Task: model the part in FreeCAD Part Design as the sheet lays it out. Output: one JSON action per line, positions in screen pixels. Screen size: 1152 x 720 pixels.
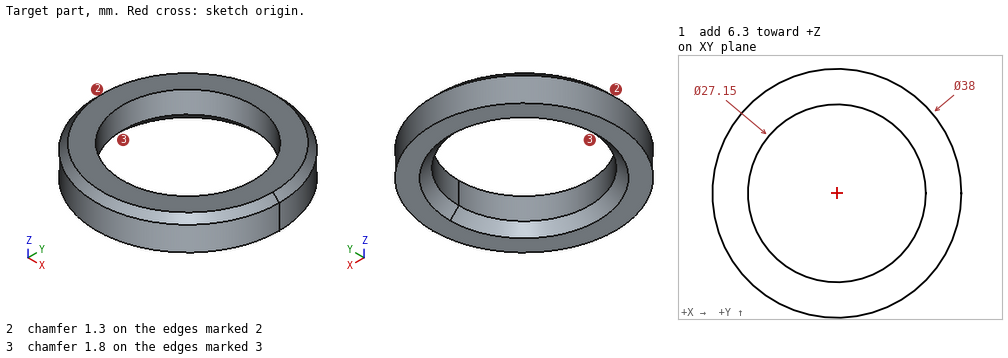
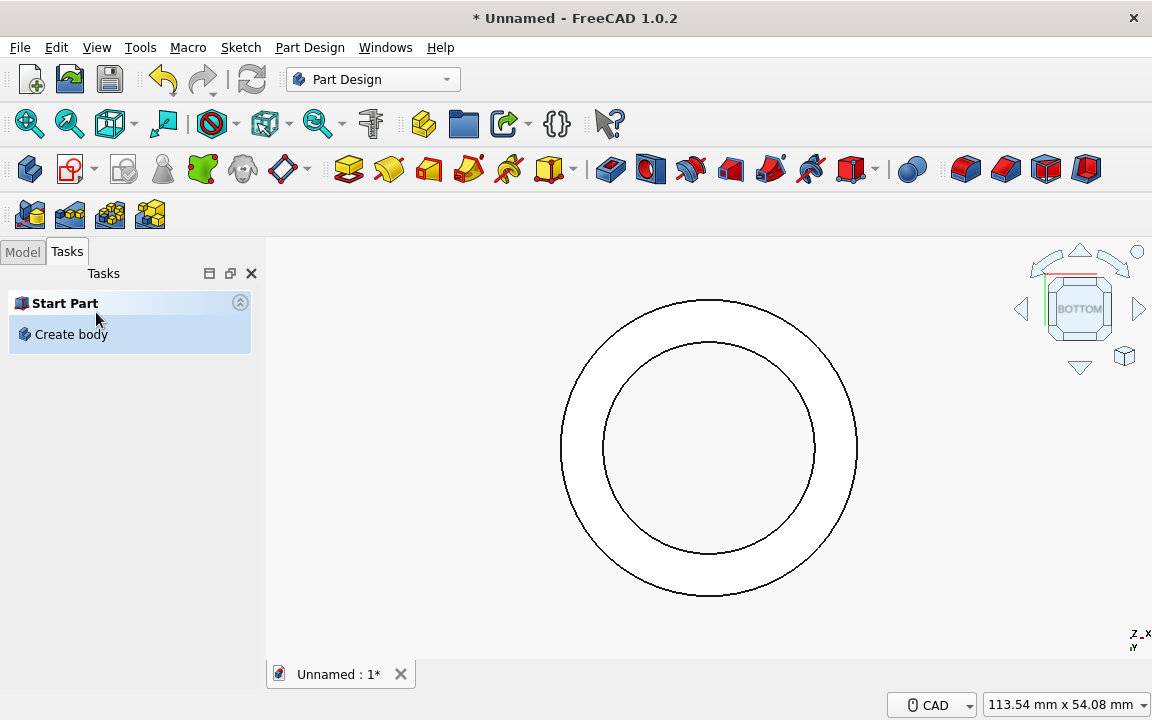
{"action": "left_click", "coordinate": [676, 548]}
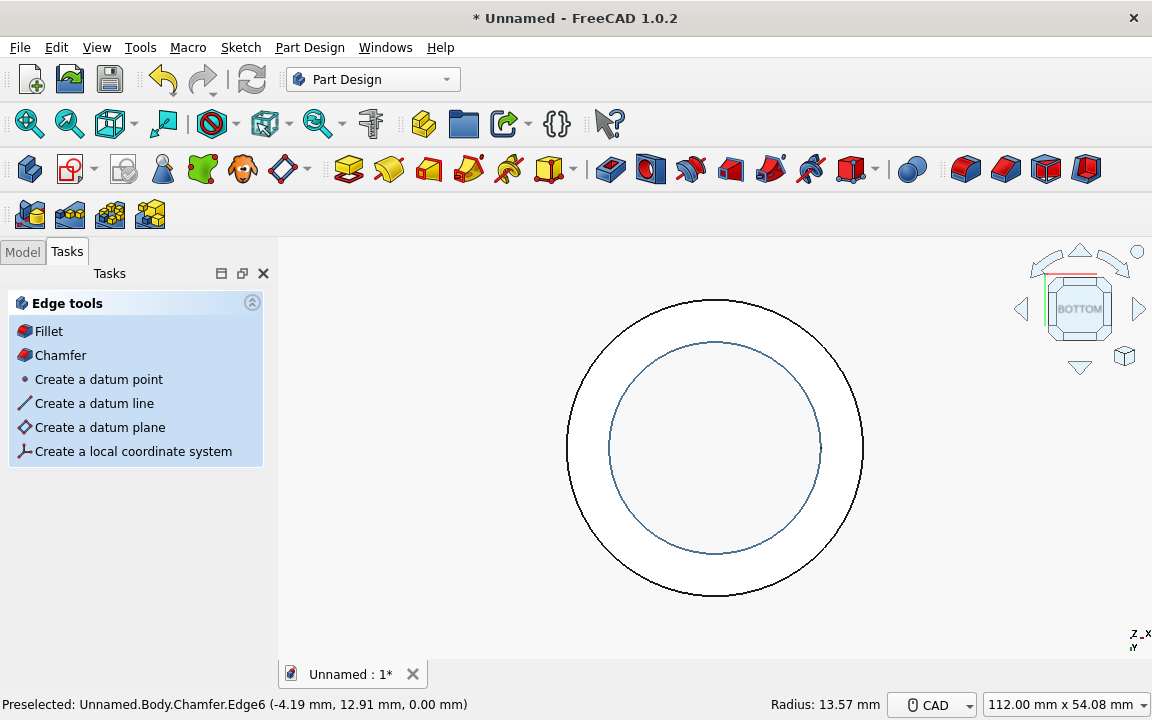
{"action": "left_click", "coordinate": [1006, 170]}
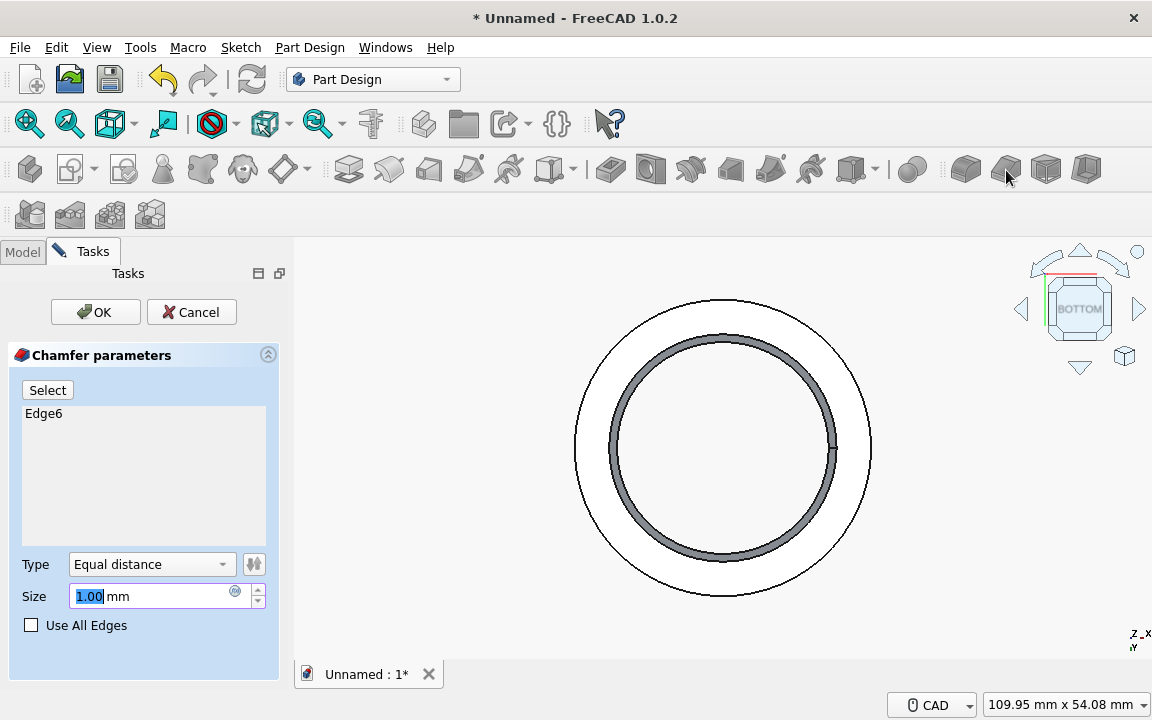
{"action": "type", "text": "1.8"}
{"action": "key", "text": "Tab"}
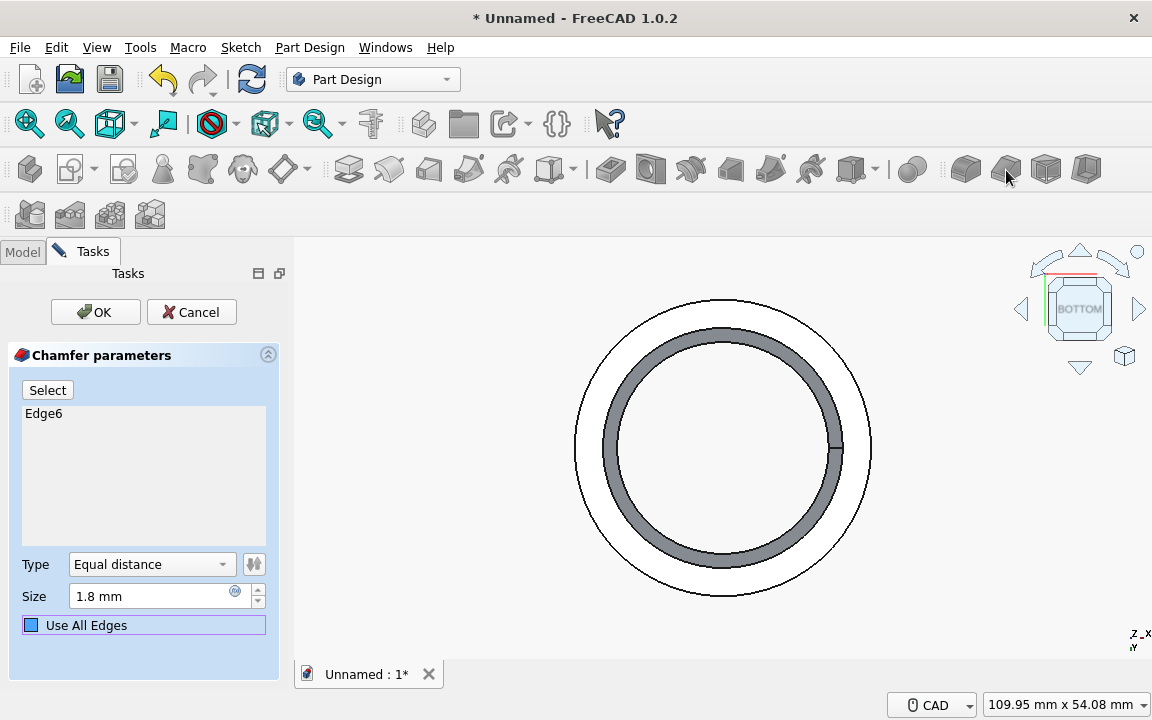
{"action": "left_click", "coordinate": [96, 312]}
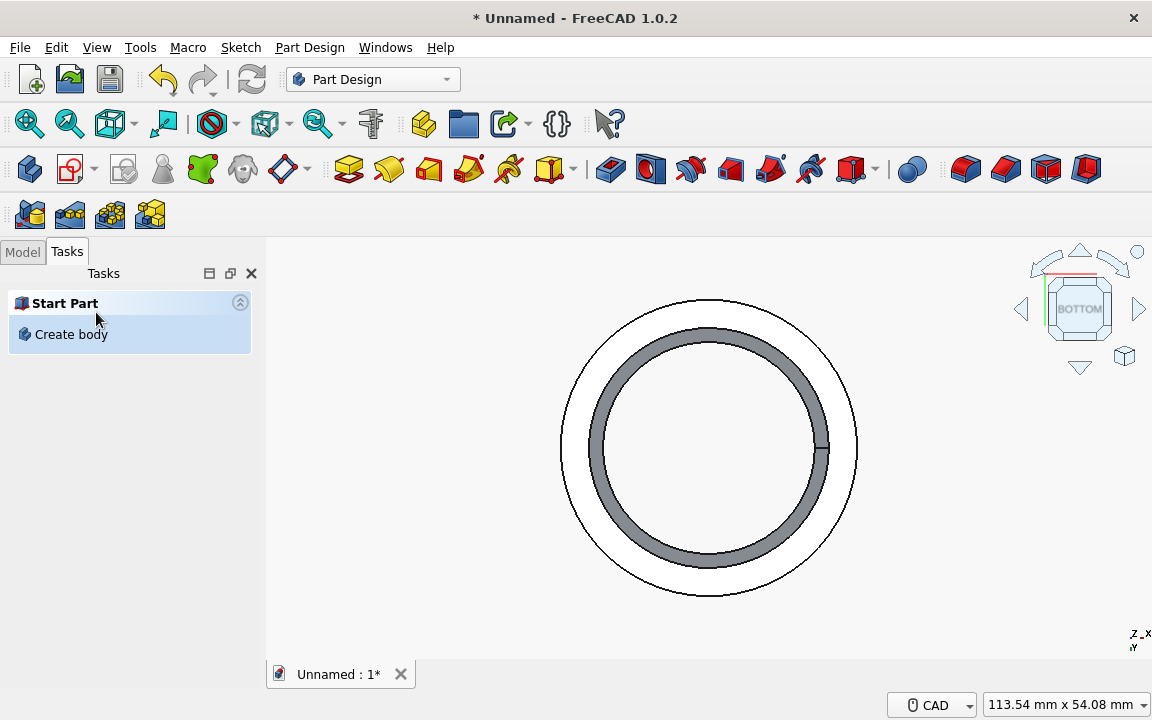
{"action": "key", "text": "0"}